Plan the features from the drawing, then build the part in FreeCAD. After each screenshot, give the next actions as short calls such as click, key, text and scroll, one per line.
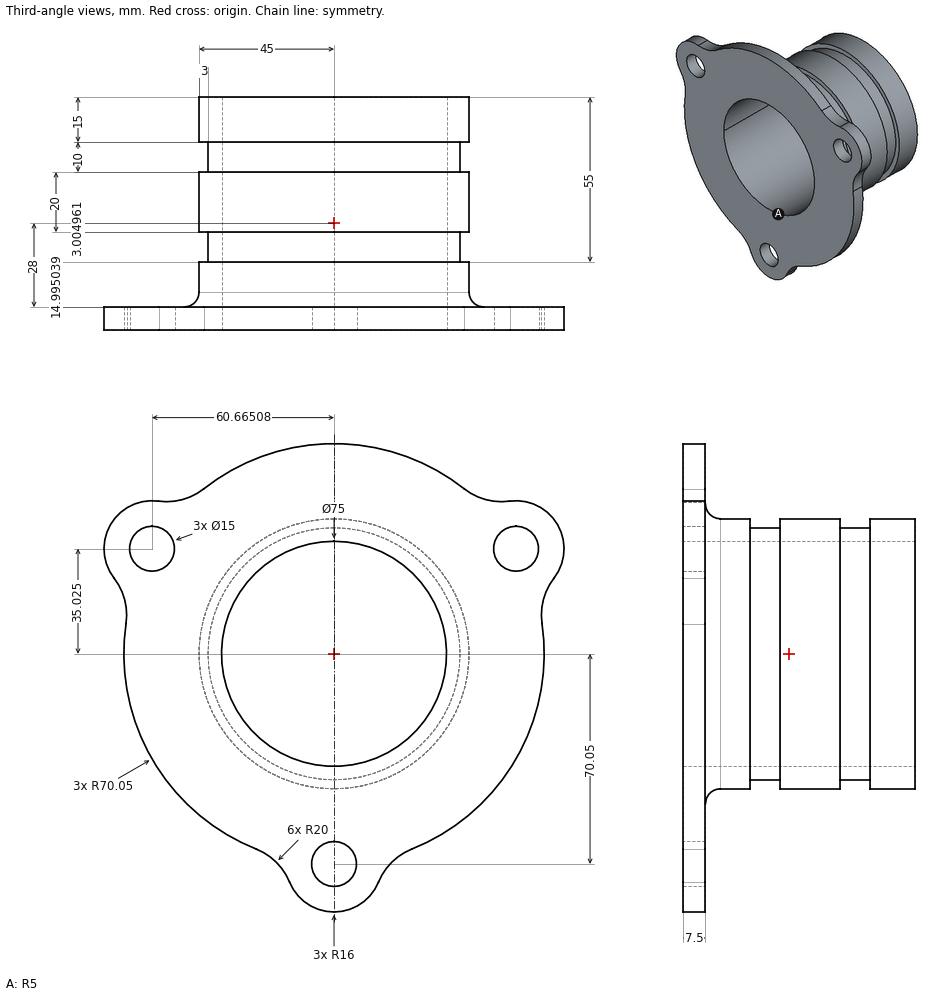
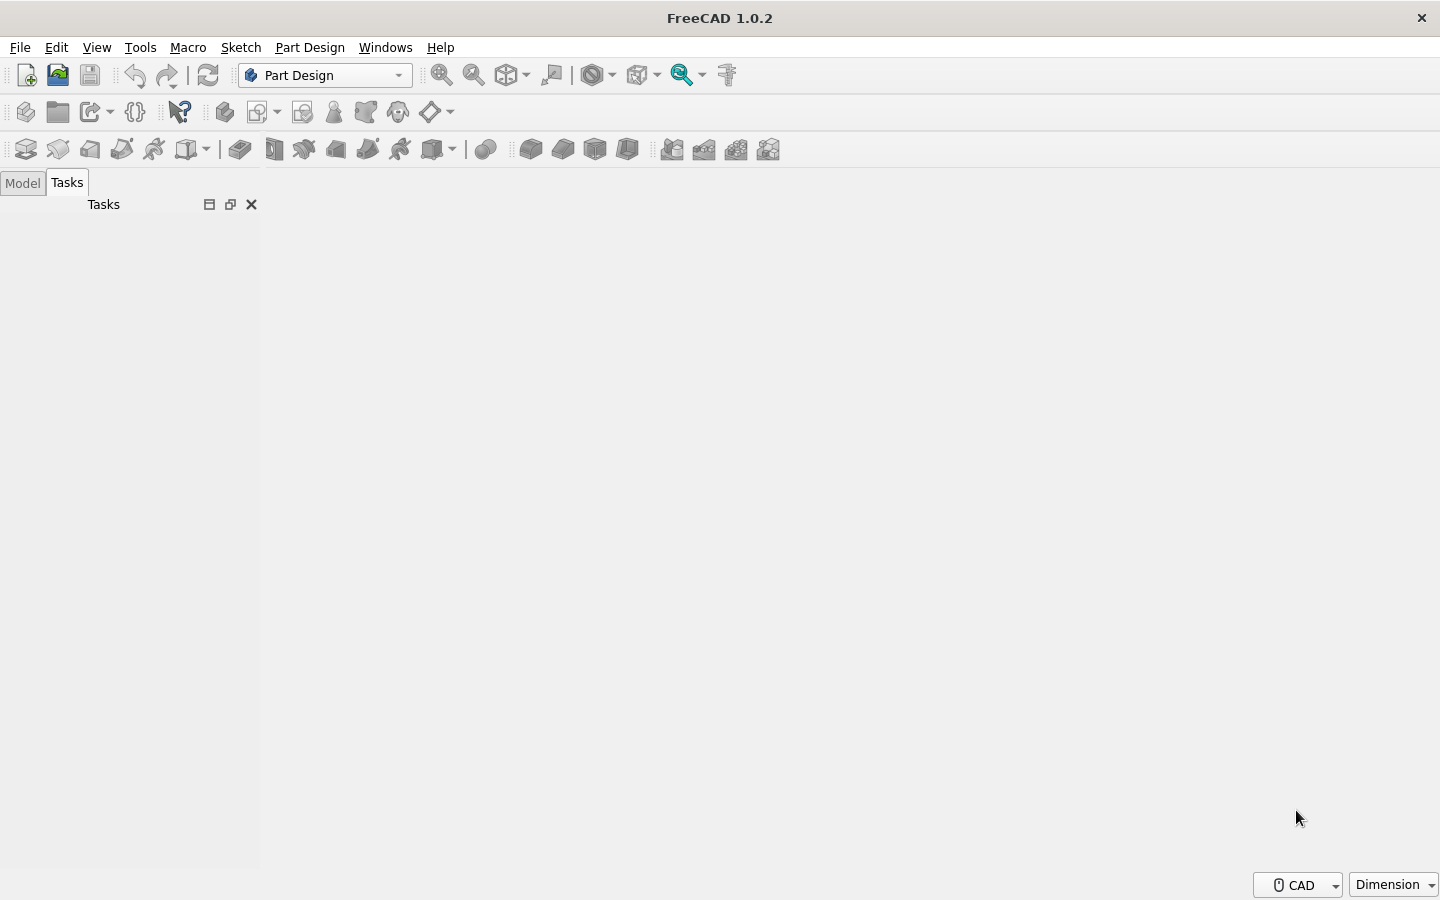
key(ctrl+n)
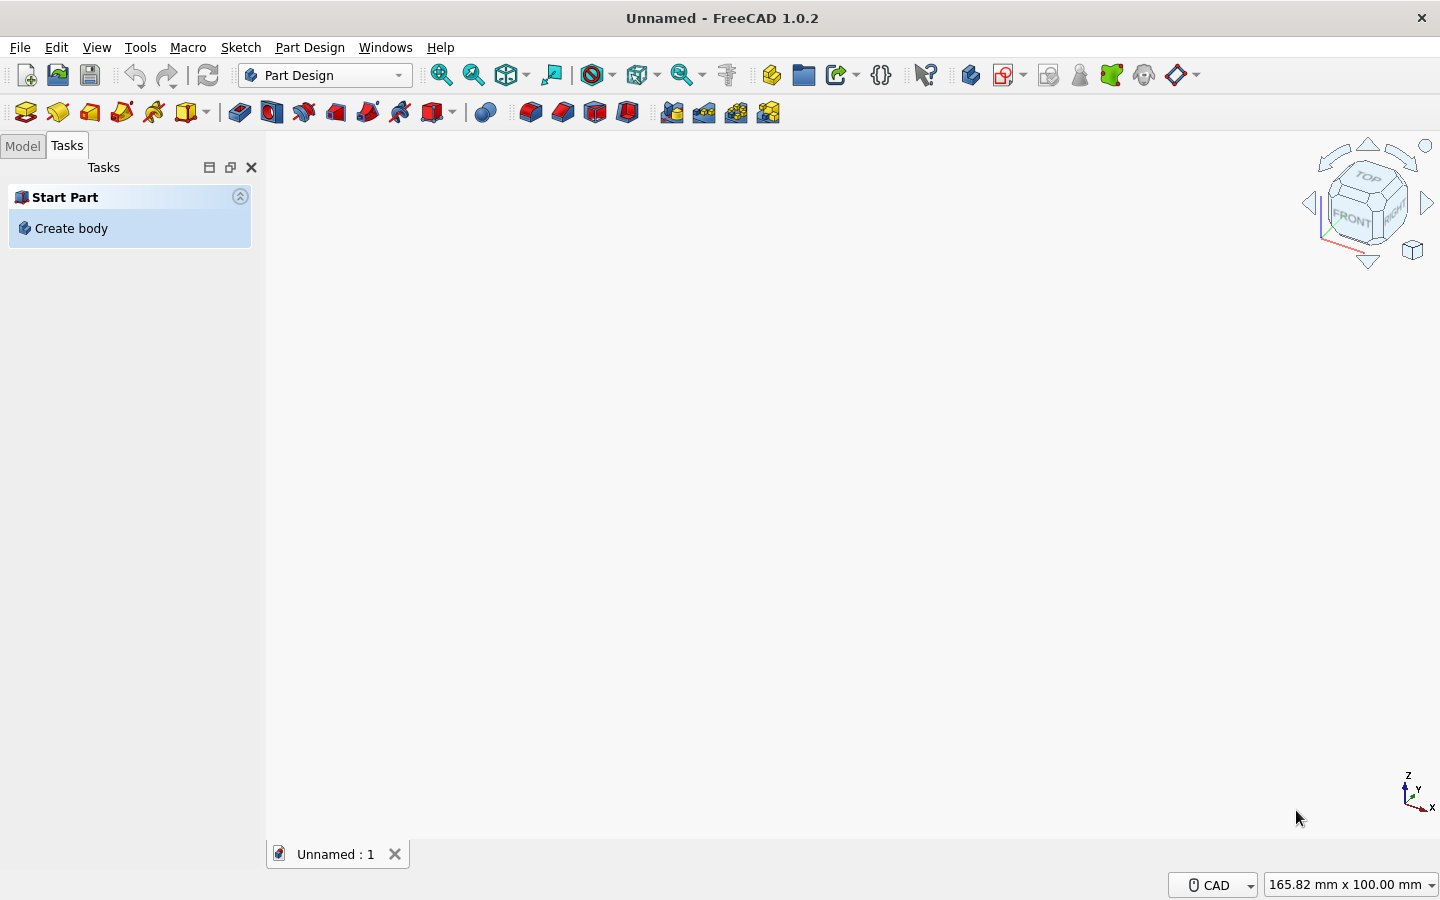
click(1004, 76)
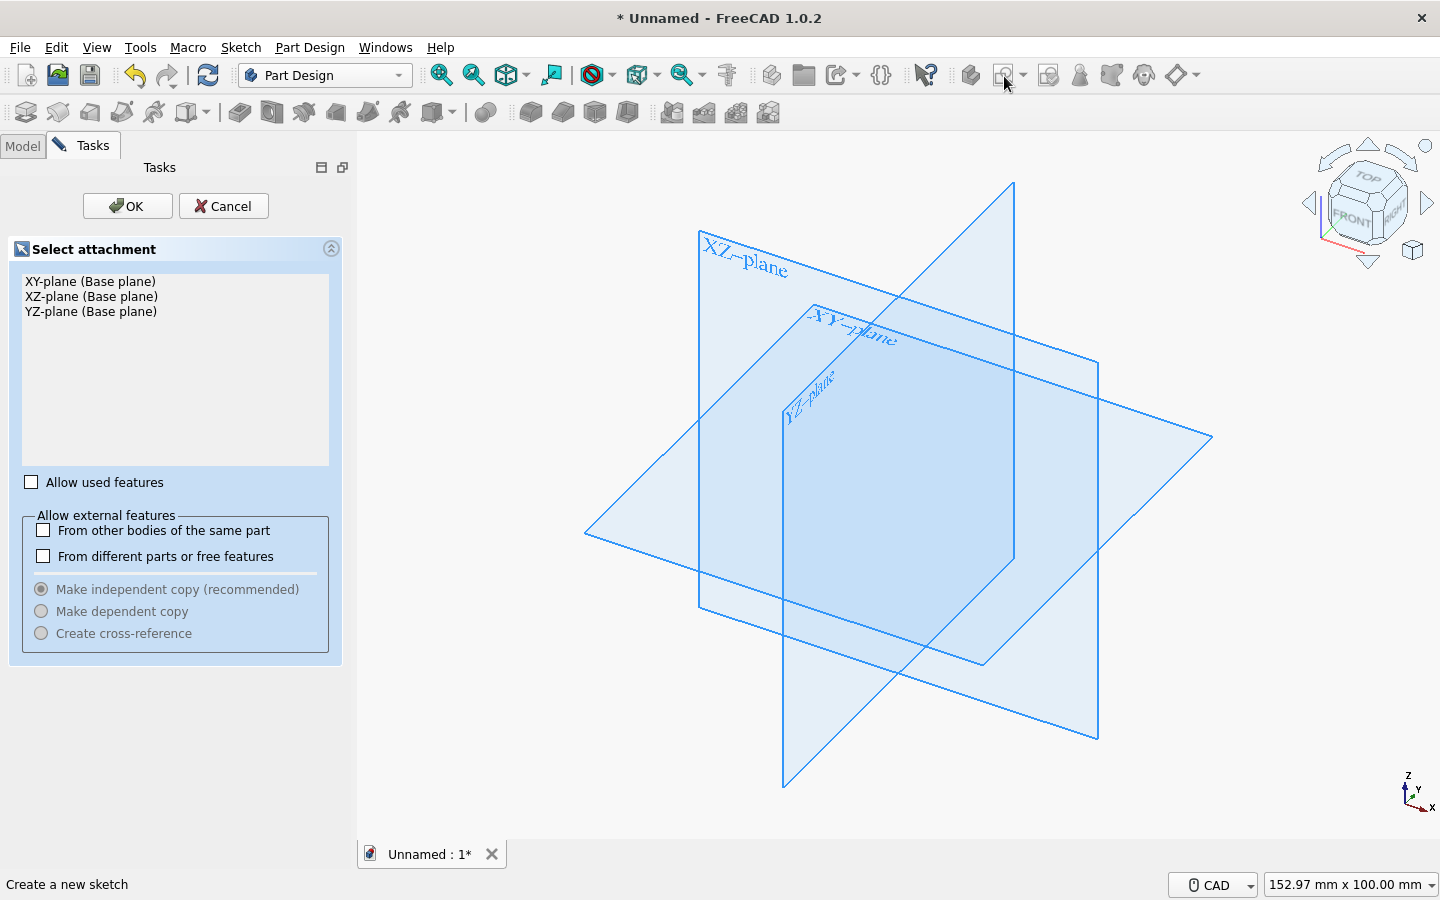
click(82, 282)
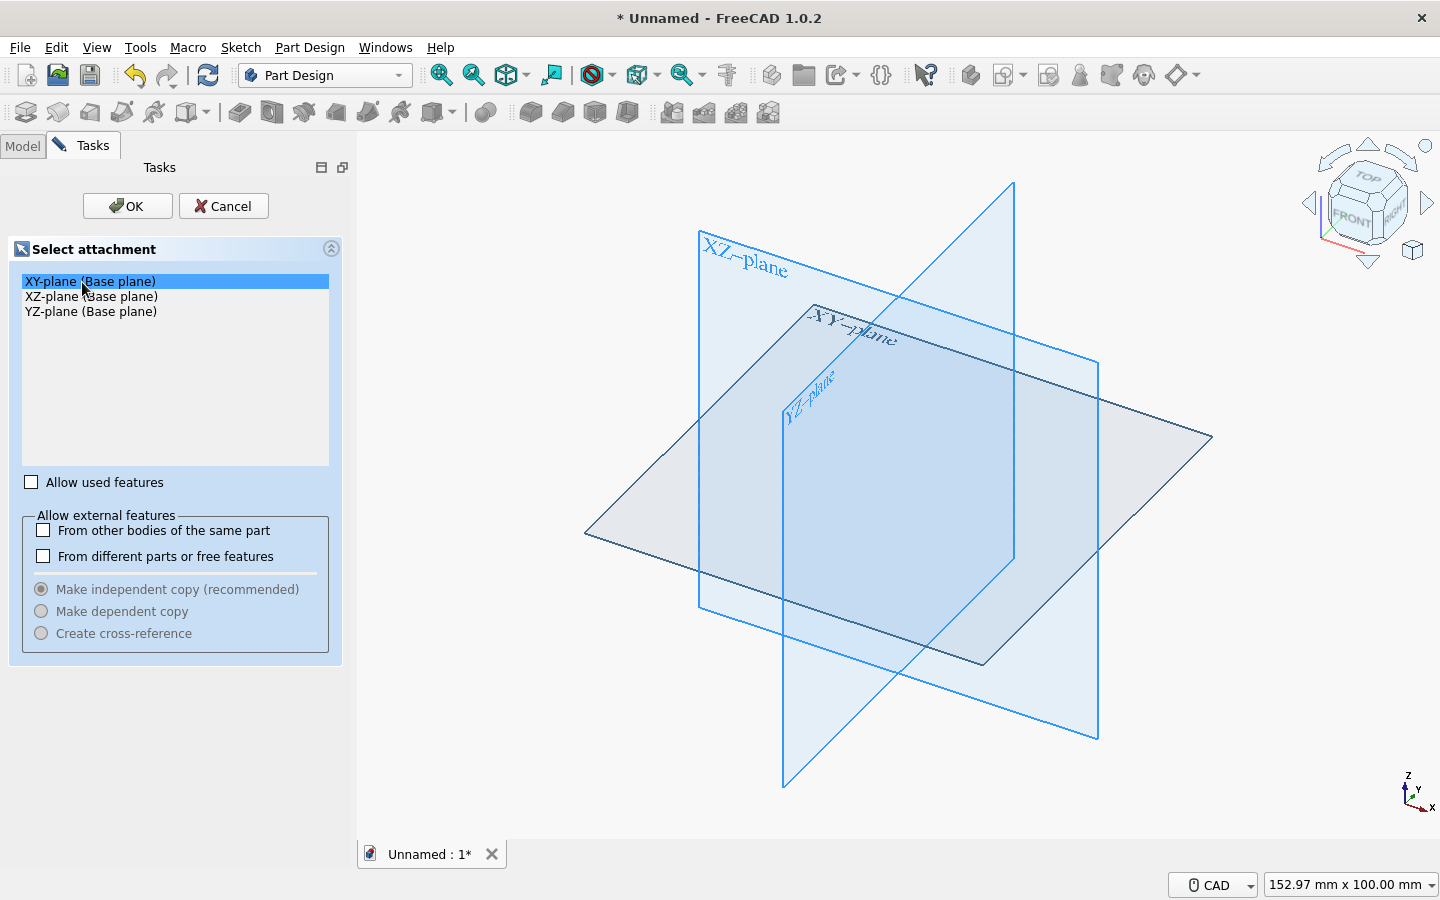
click(128, 206)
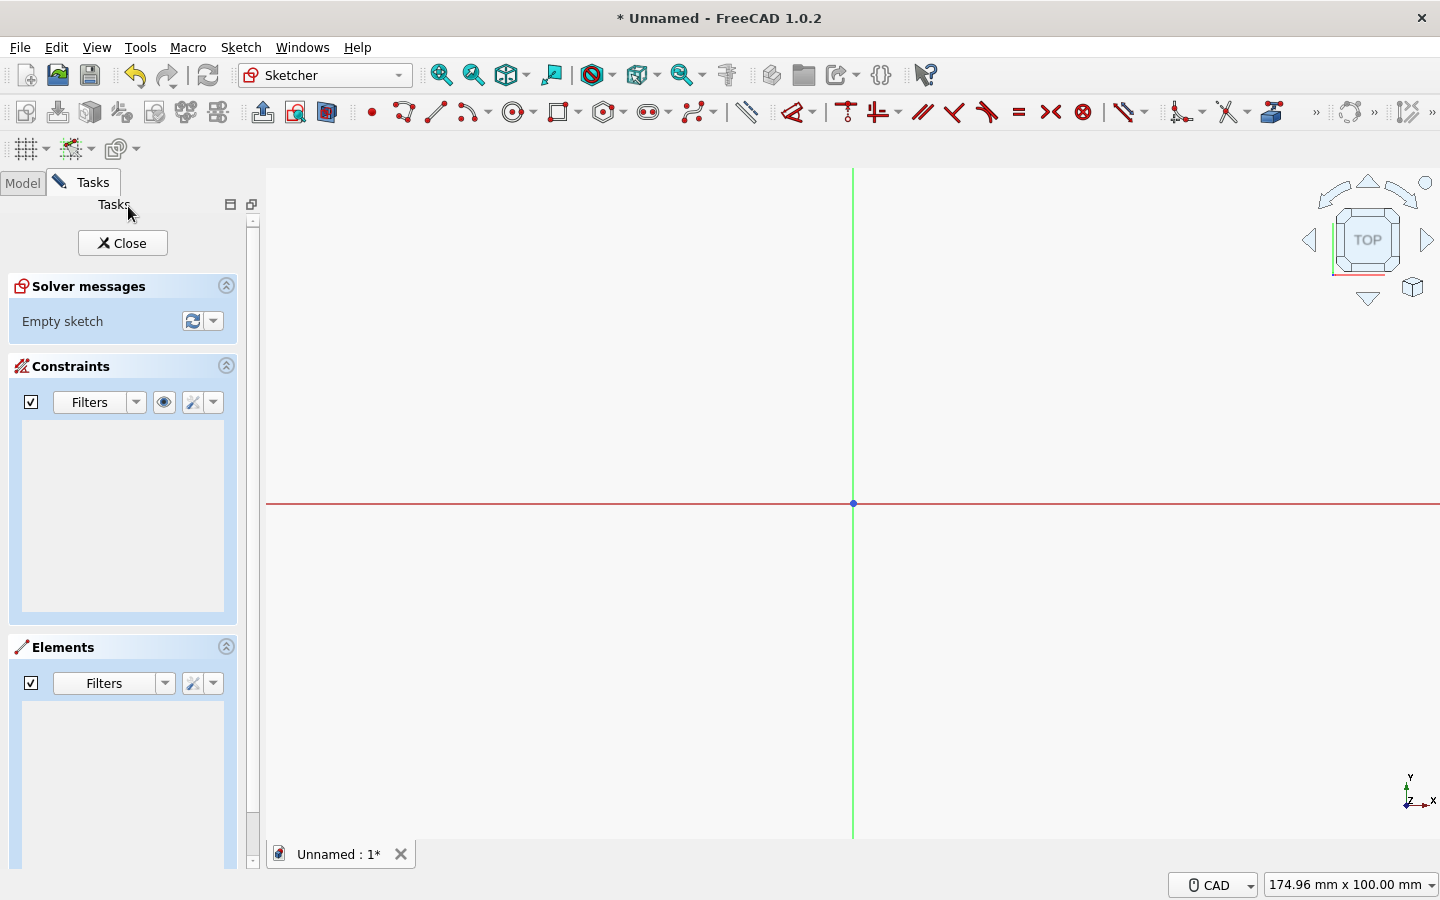
key(g)
key(m)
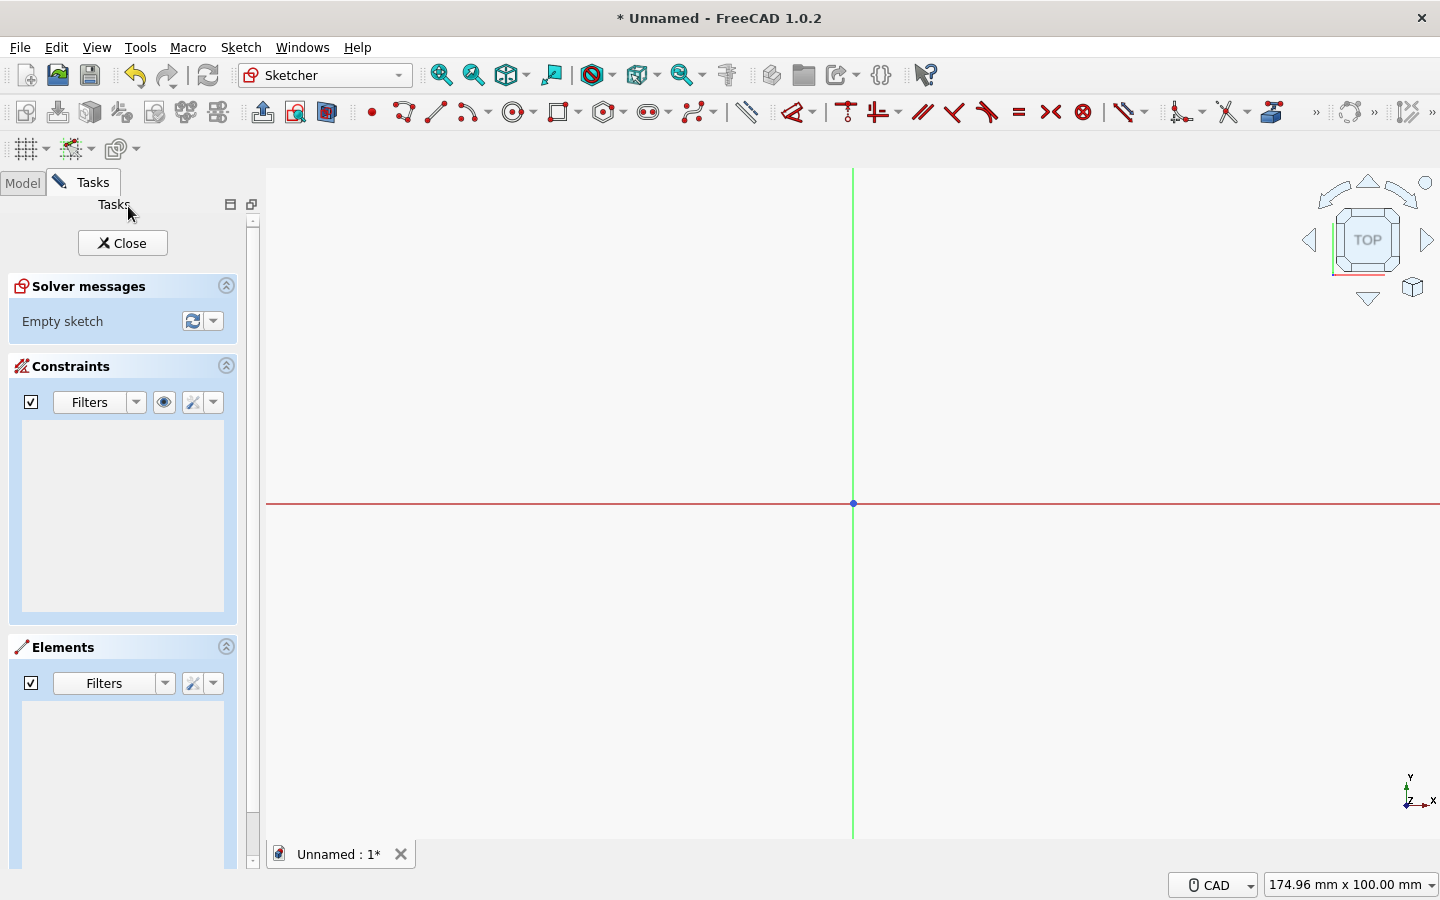
click(853, 591)
click(844, 222)
click(551, 222)
click(551, 322)
click(571, 322)
click(571, 389)
click(551, 389)
click(551, 524)
click(571, 524)
click(571, 591)
click(853, 592)
key(Escape)
key(Escape)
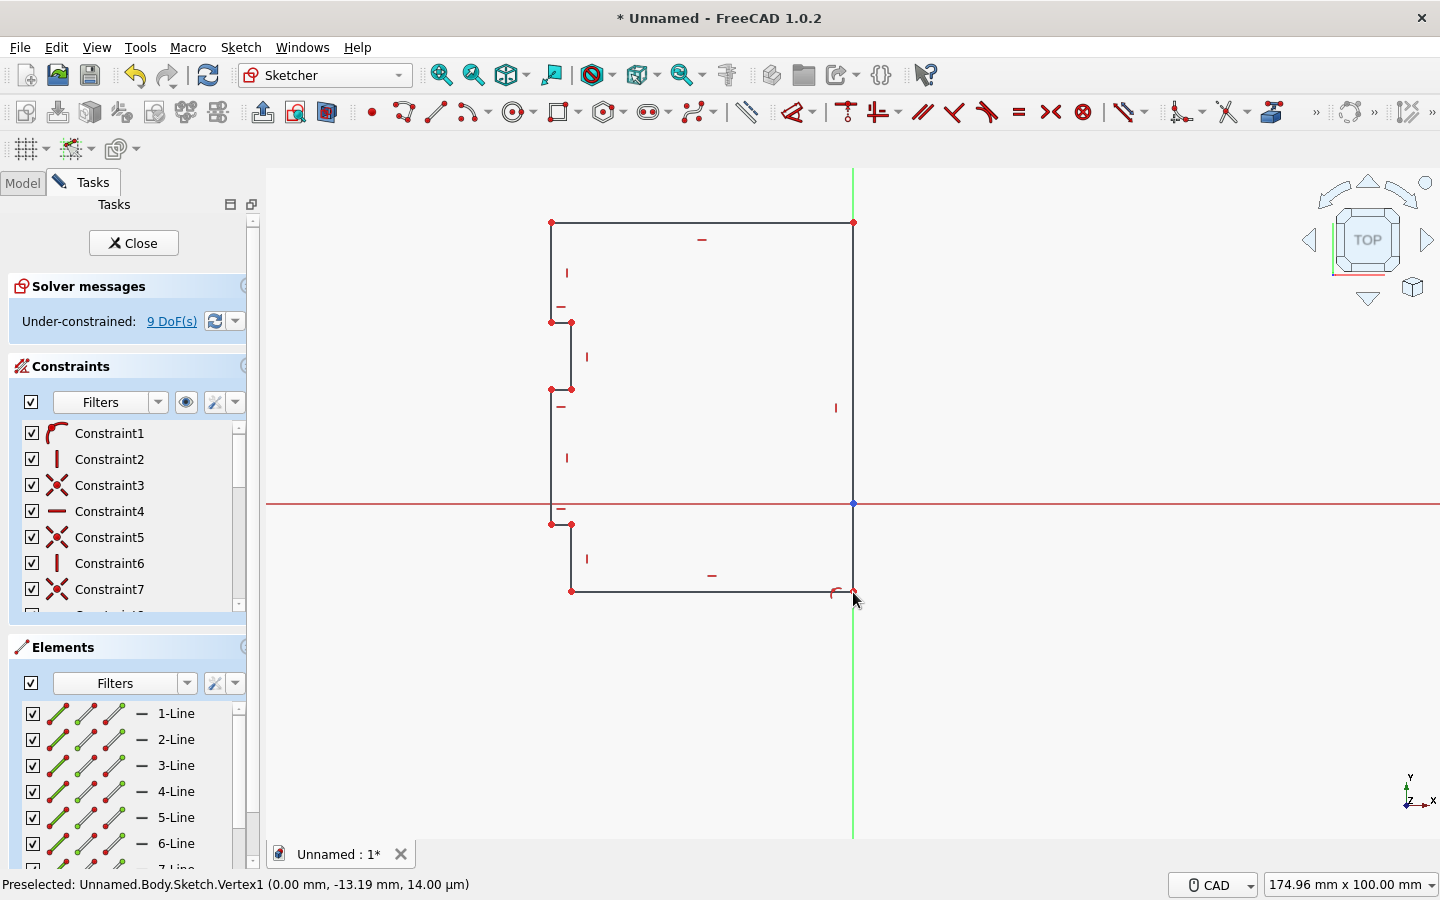
key(d)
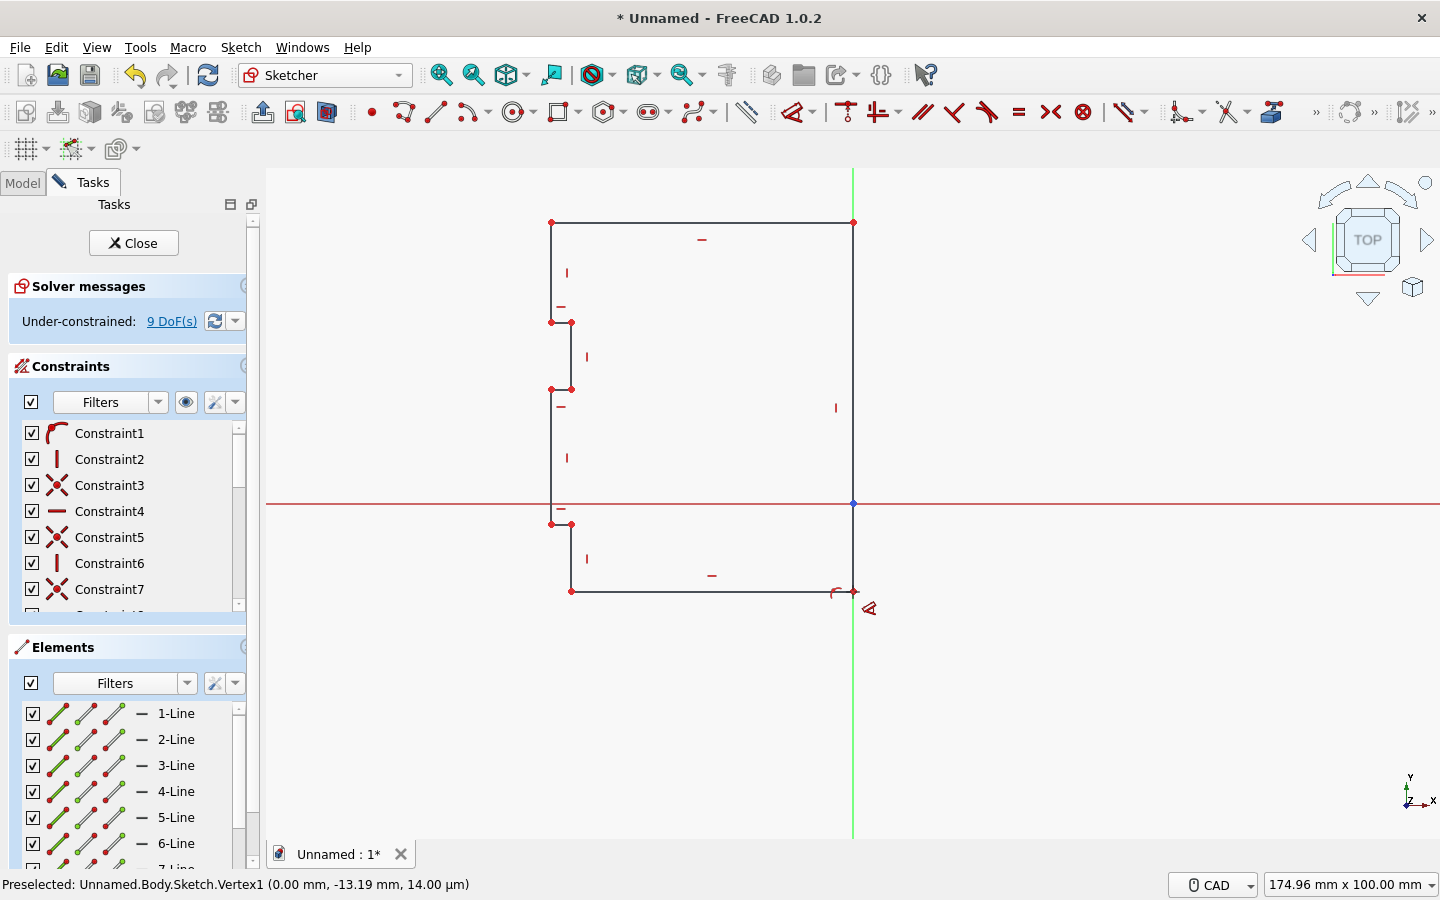
scroll(561, 323, up, 4)